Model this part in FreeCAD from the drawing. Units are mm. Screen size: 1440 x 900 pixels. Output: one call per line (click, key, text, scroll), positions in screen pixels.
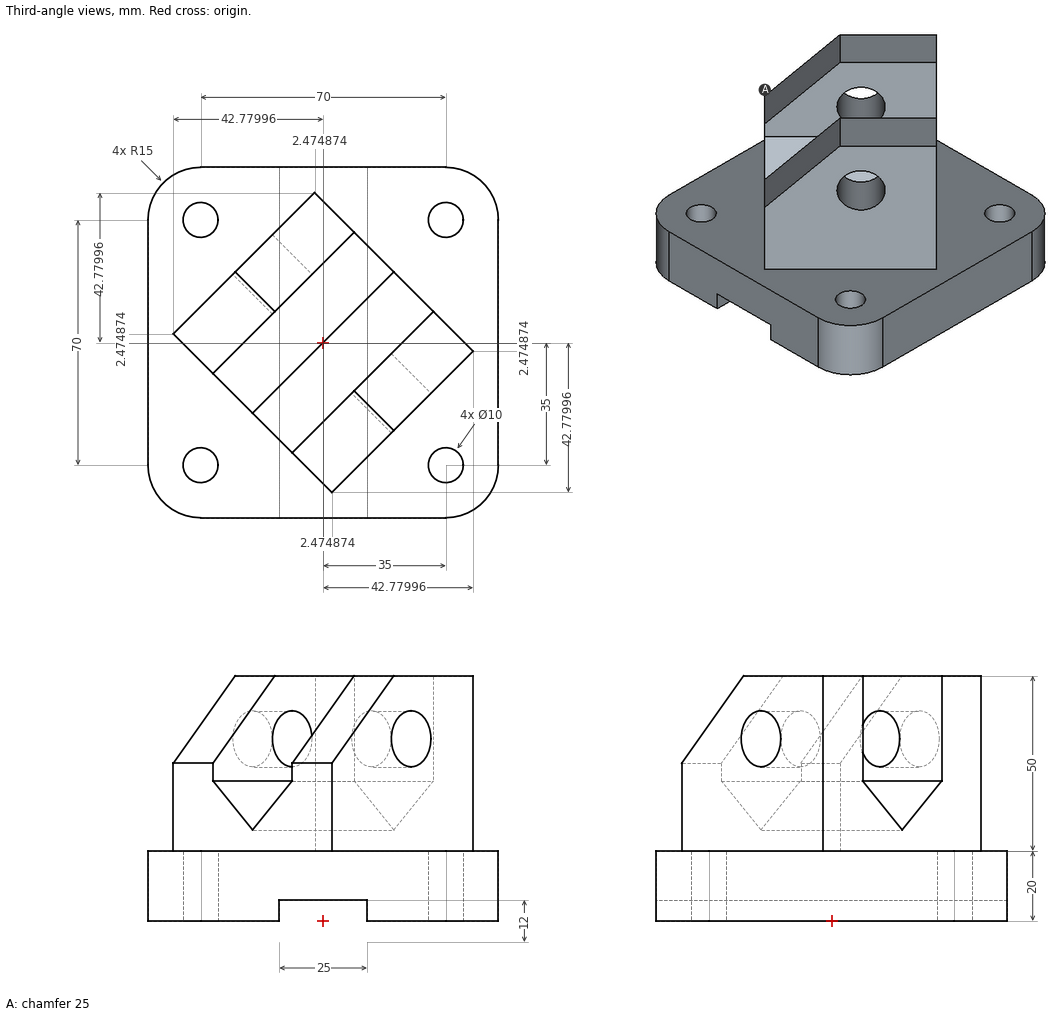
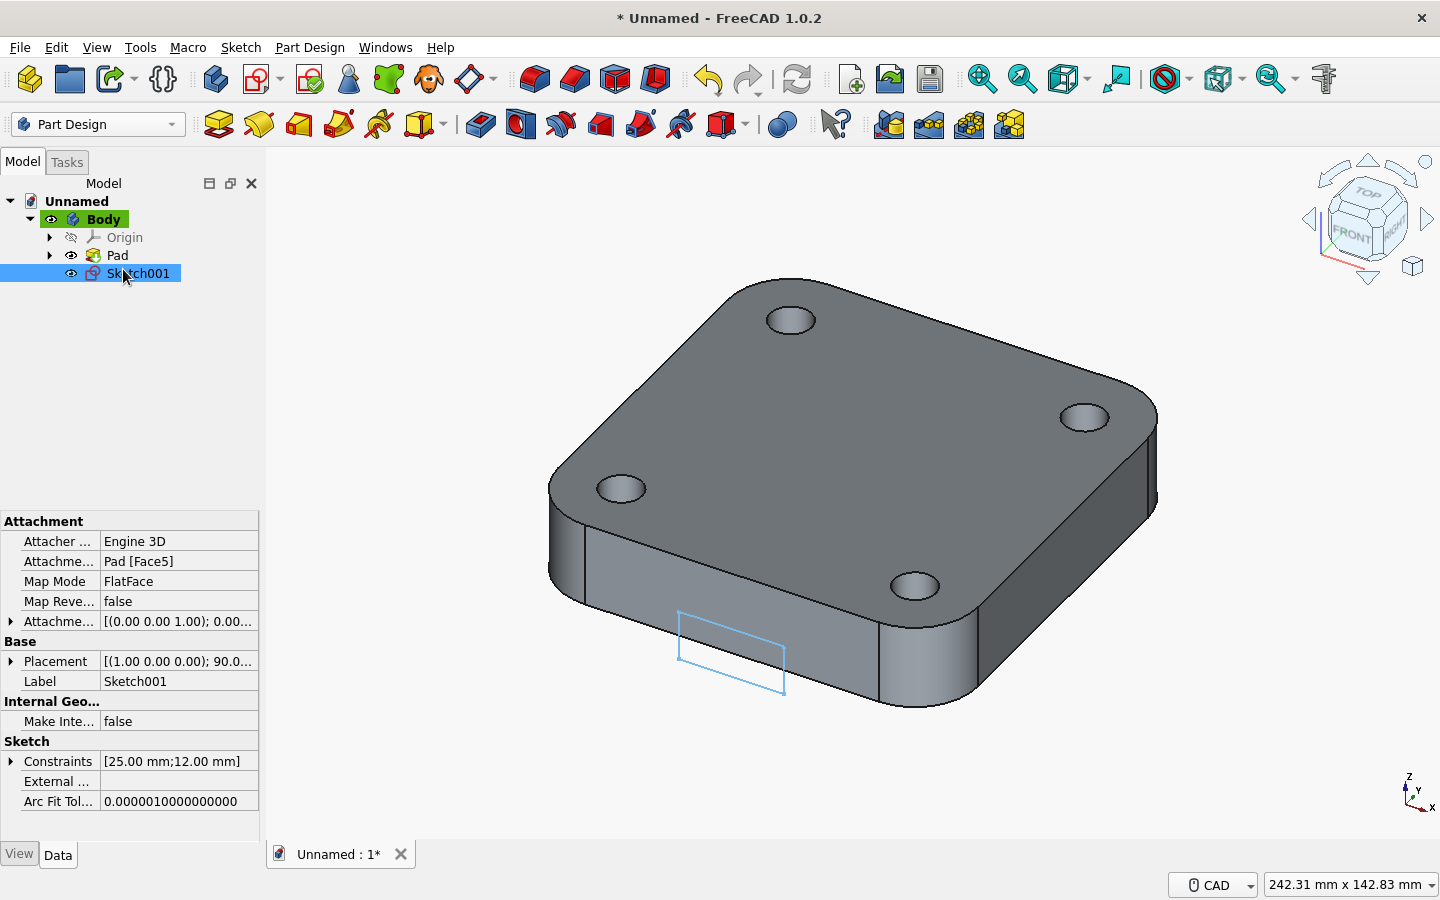
click(482, 124)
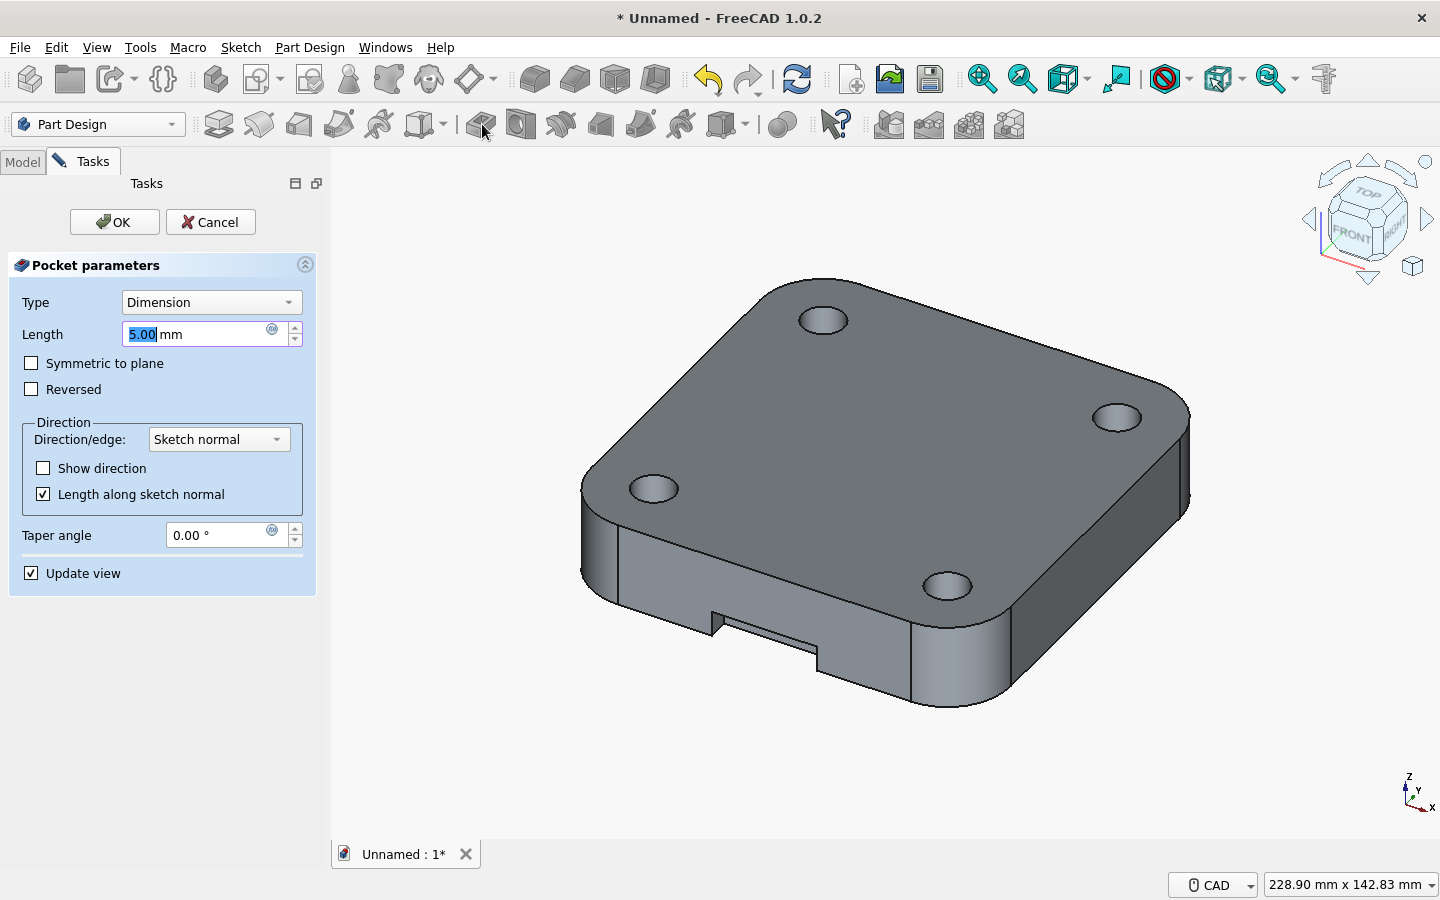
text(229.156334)
key(Tab)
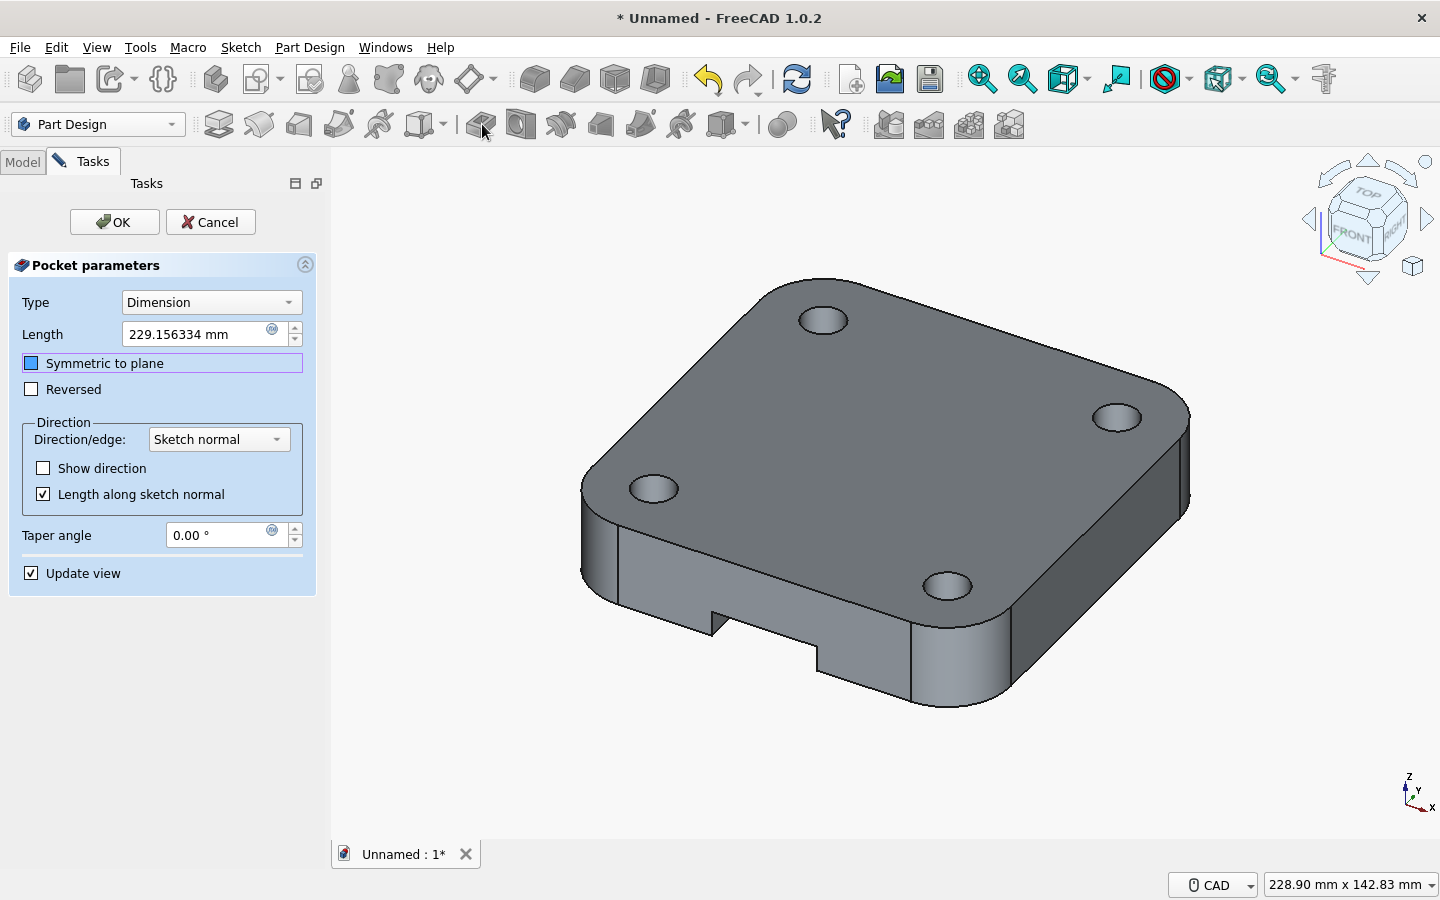
click(30, 363)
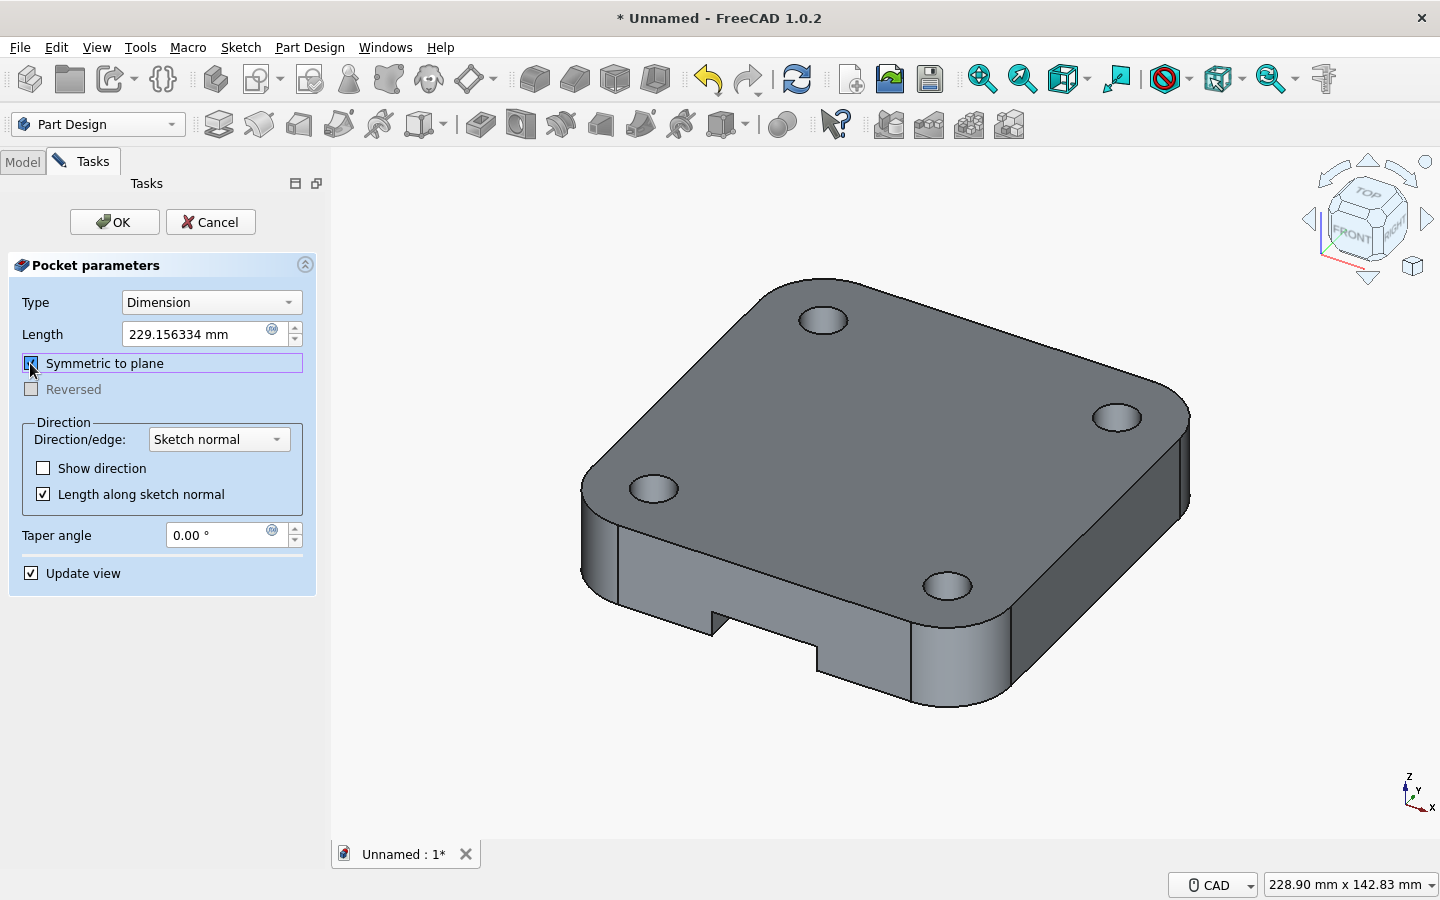
click(115, 222)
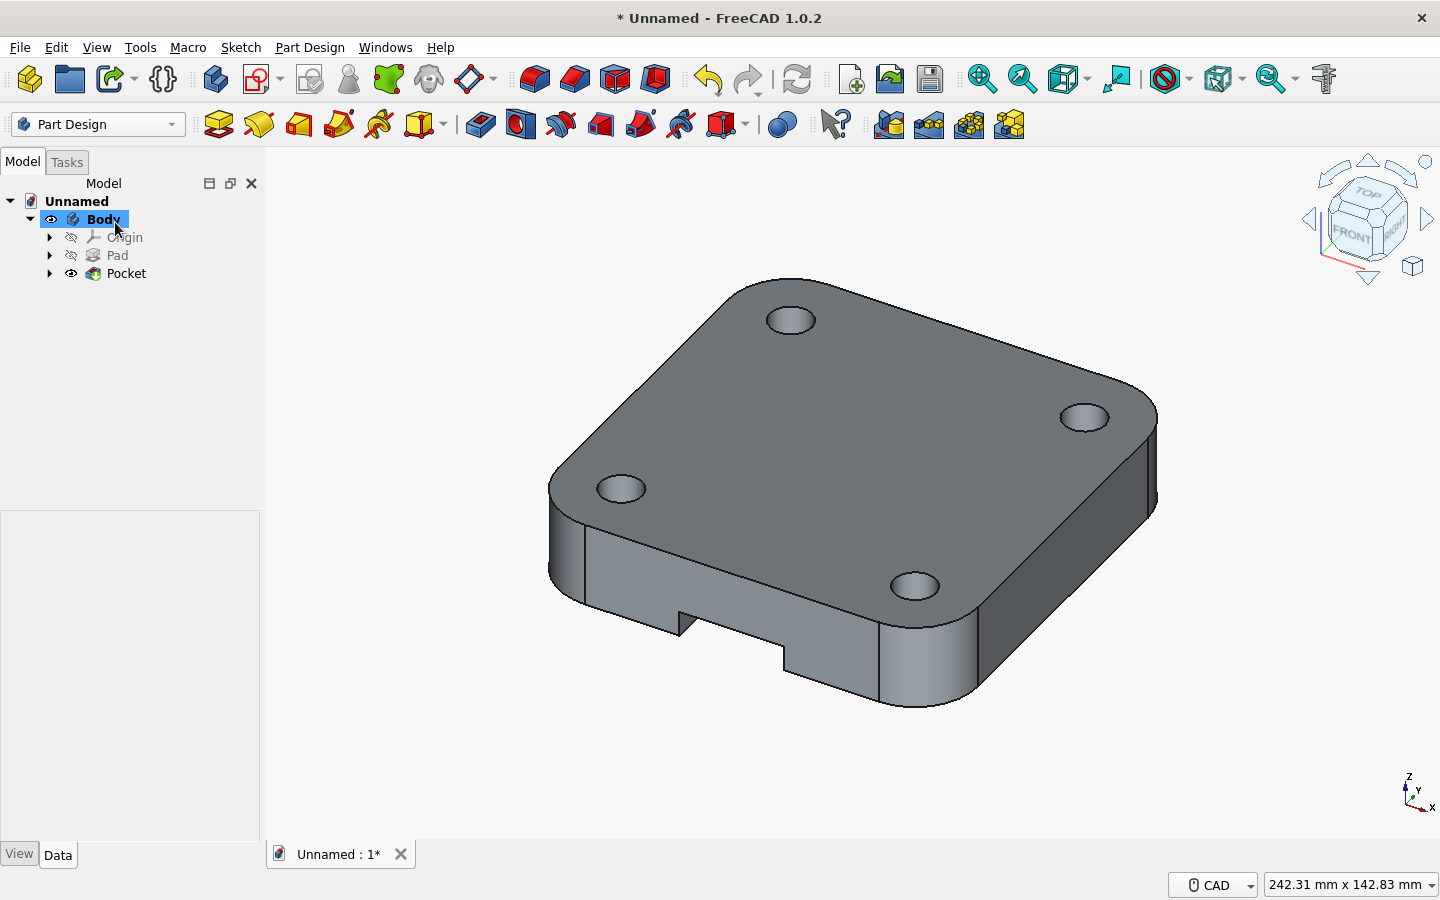
click(853, 452)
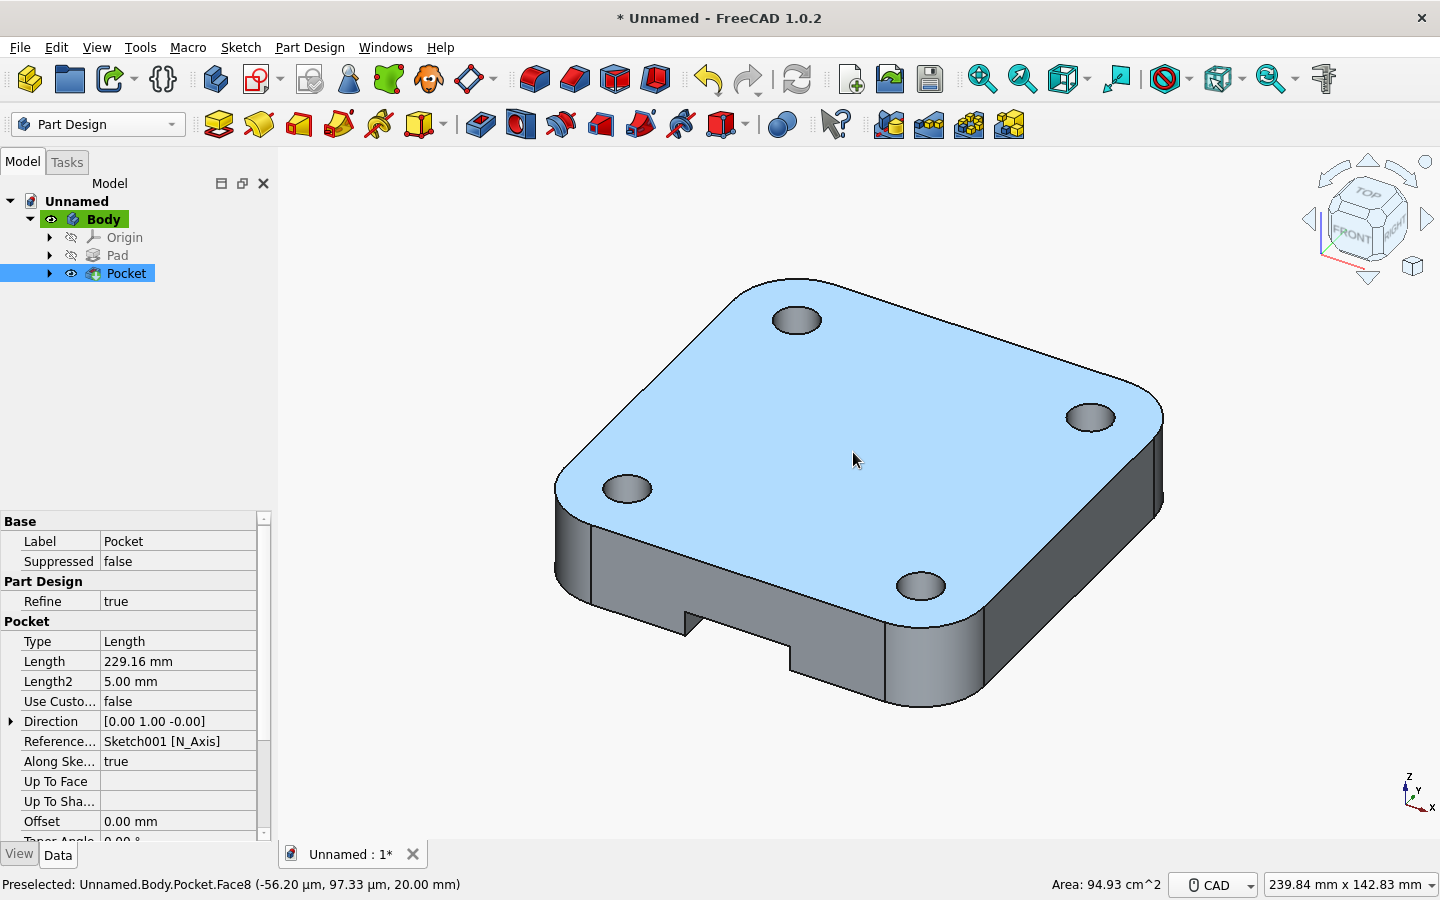
click(256, 80)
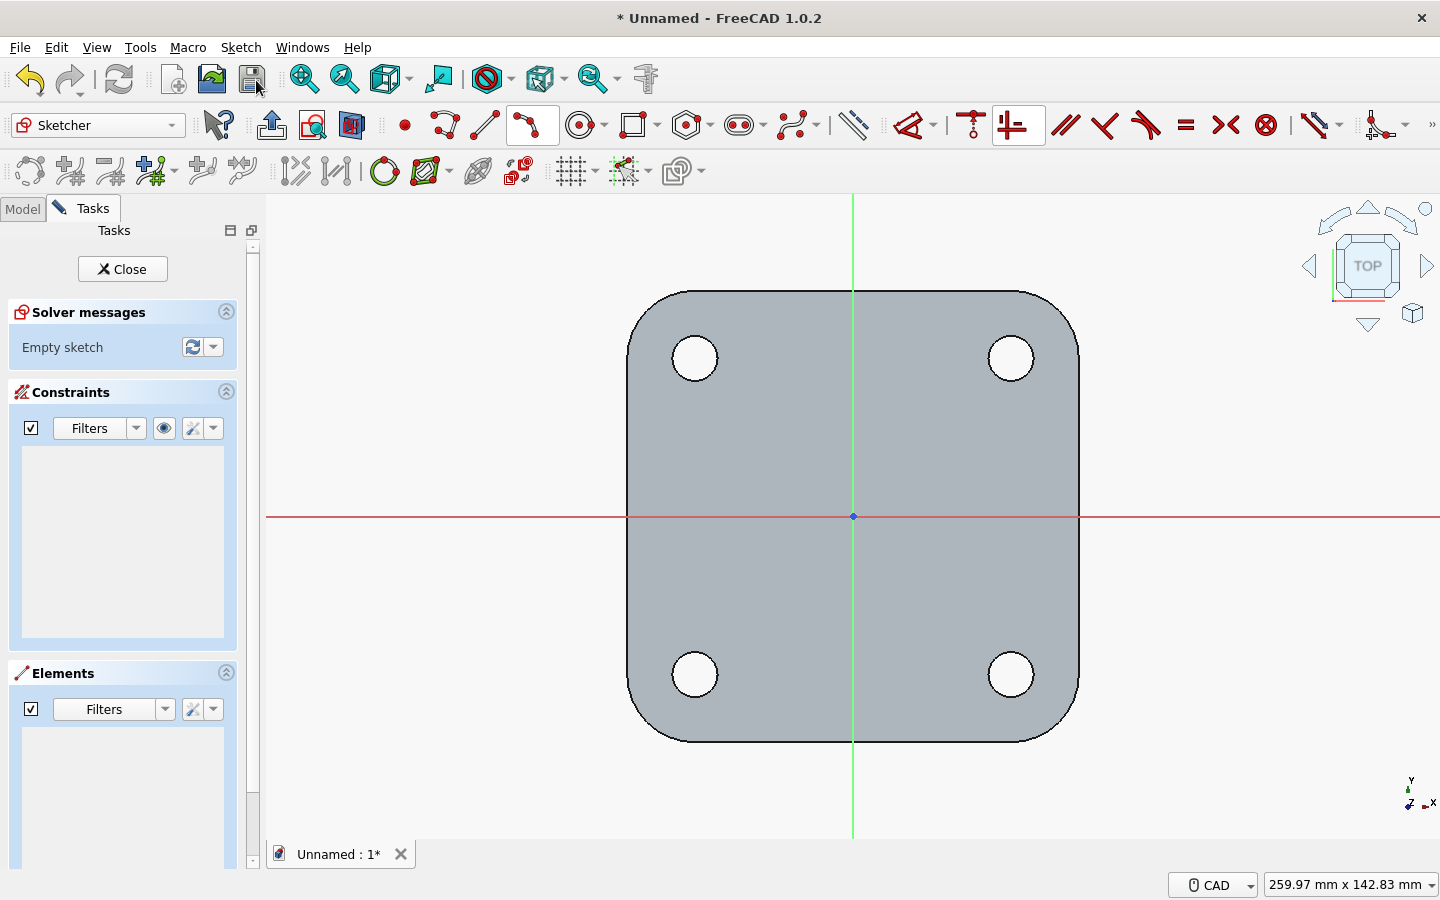
key(g)
key(m)